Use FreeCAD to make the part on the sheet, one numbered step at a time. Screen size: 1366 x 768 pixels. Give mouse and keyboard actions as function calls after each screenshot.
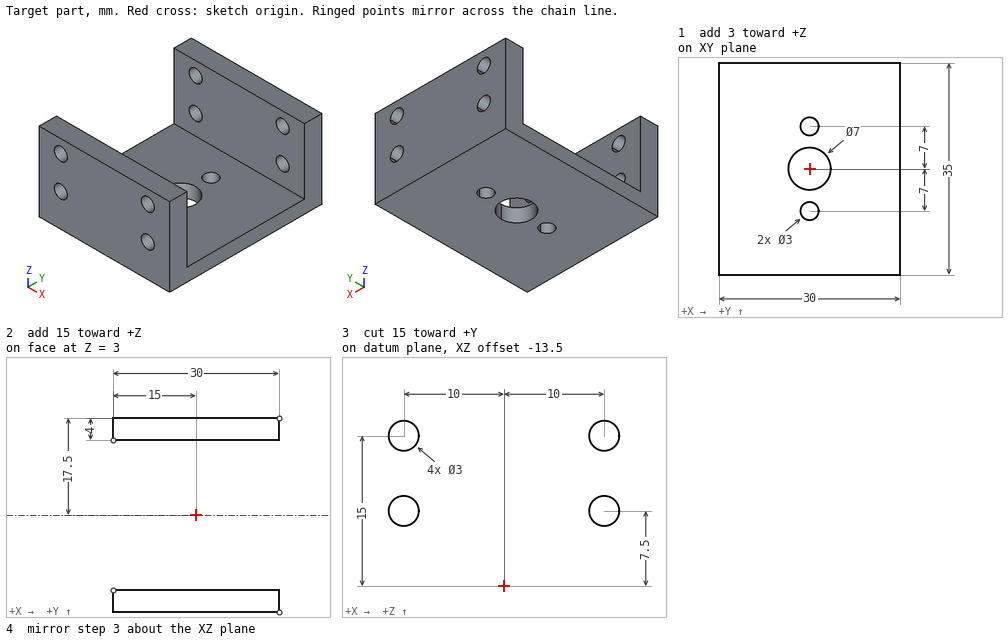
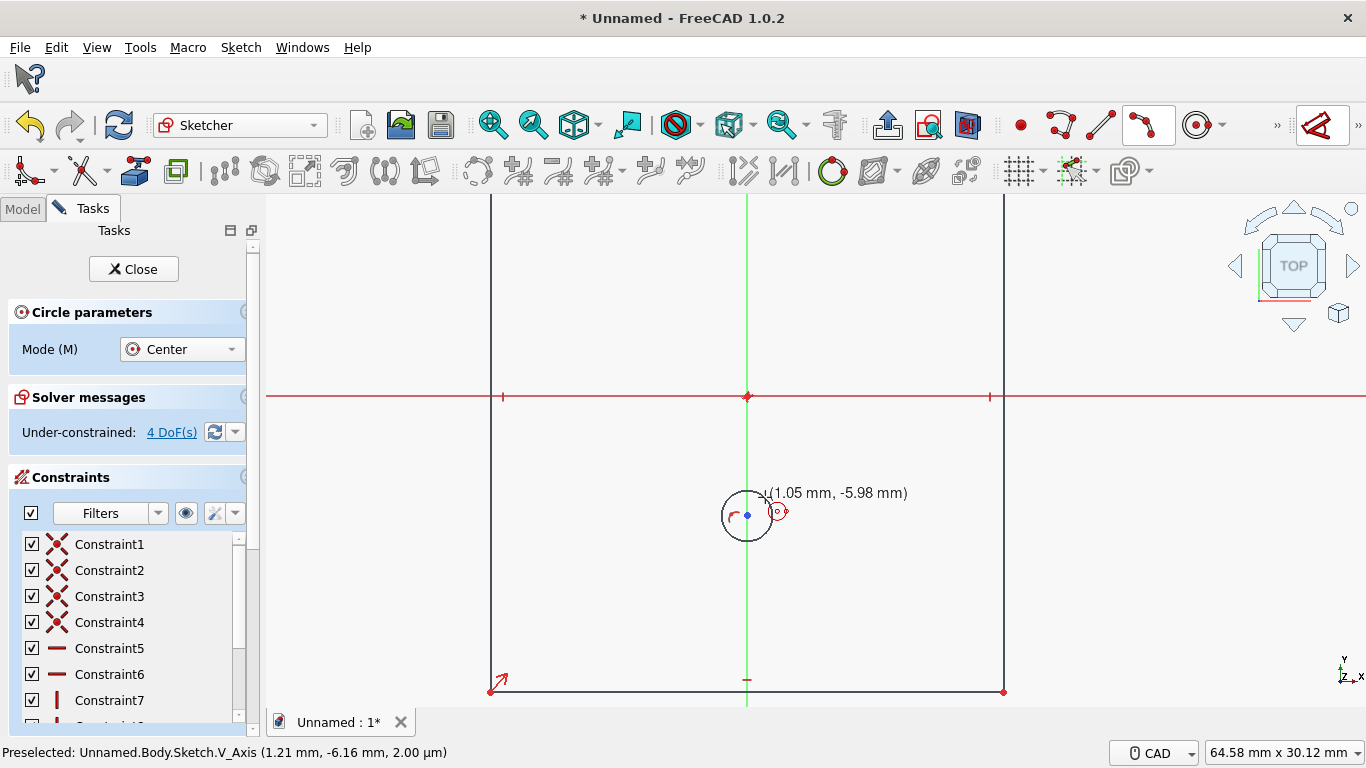
click(747, 396)
click(789, 354)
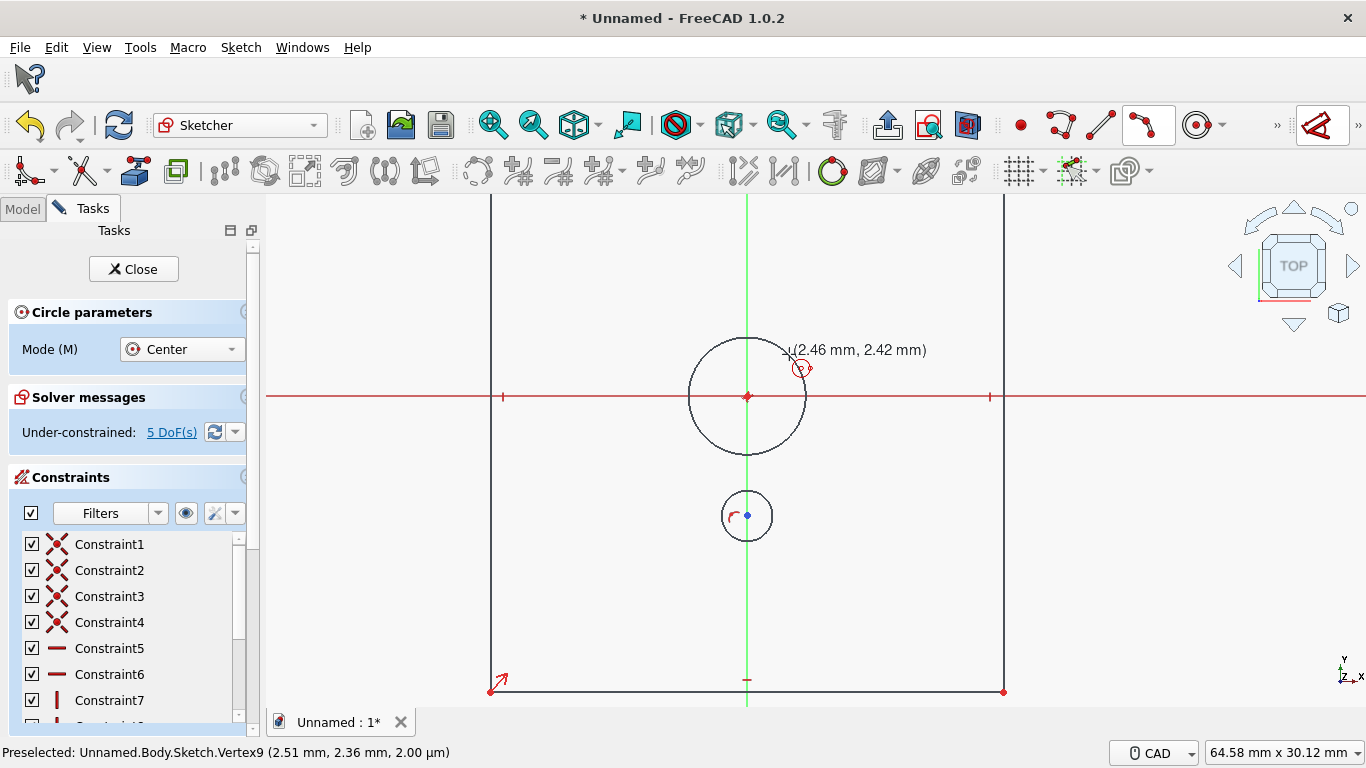
click(747, 277)
click(765, 259)
key(Escape)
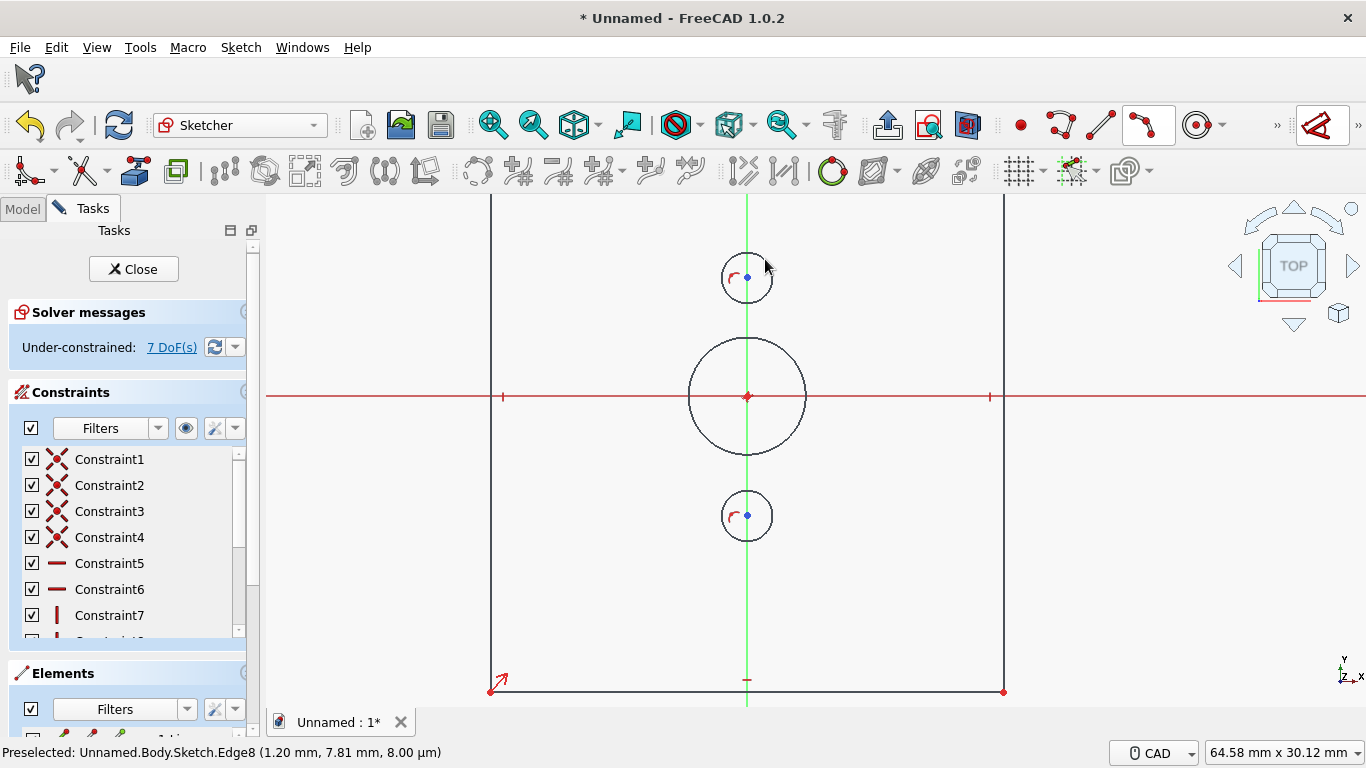
click(765, 498)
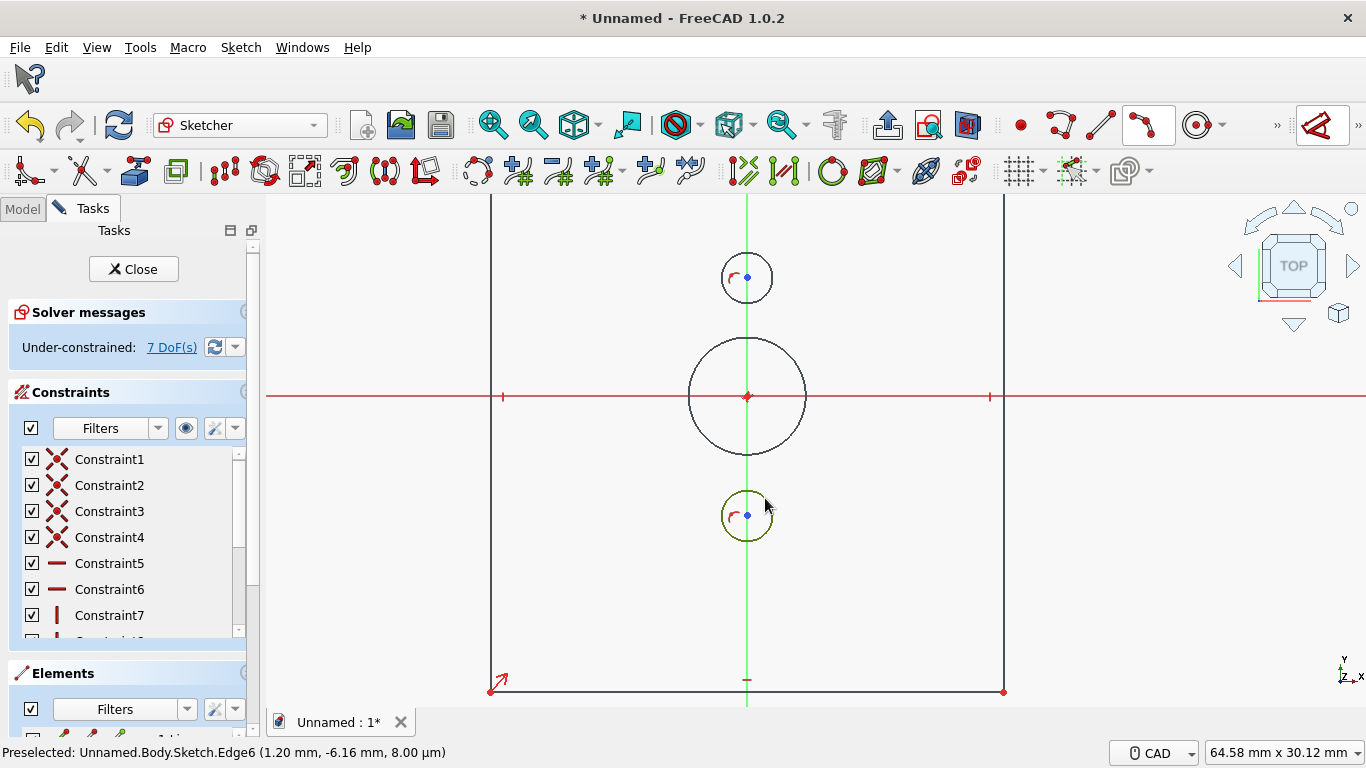
click(765, 260)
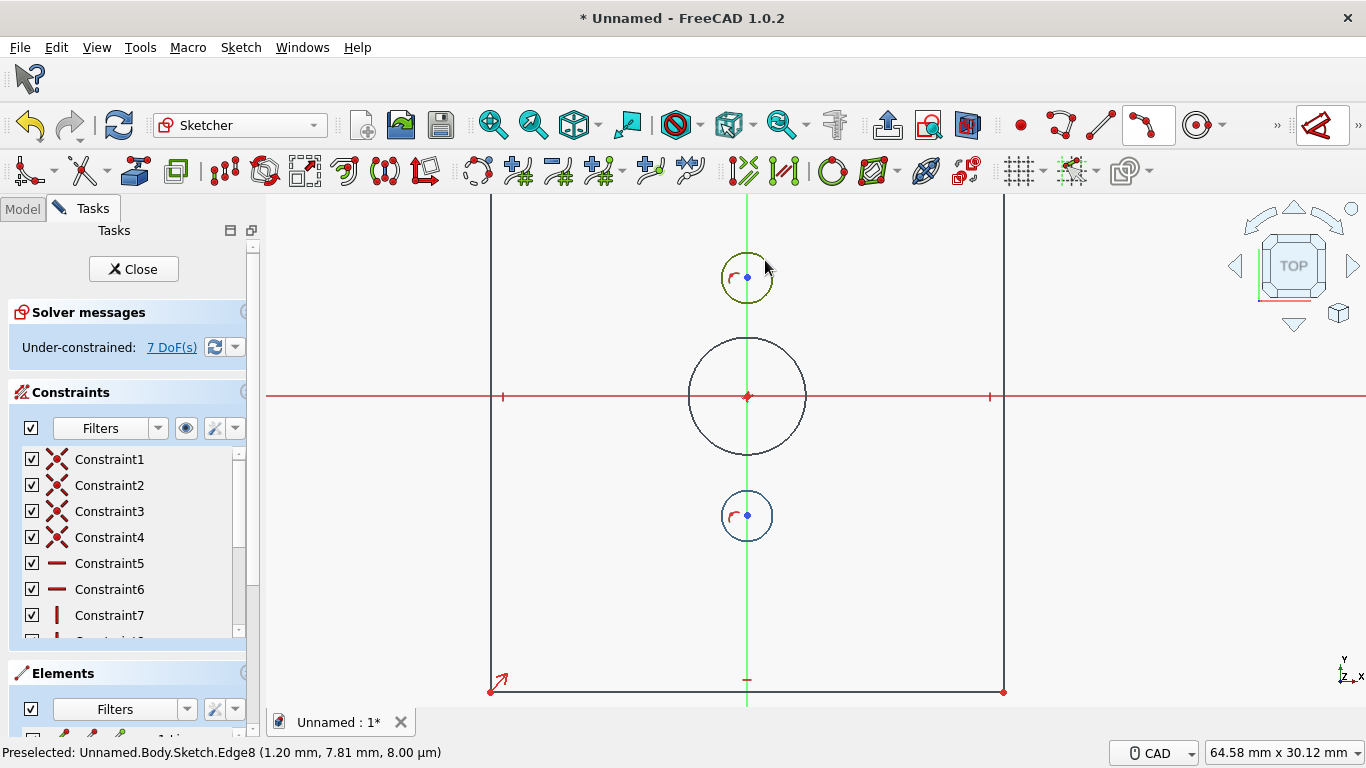
key(e)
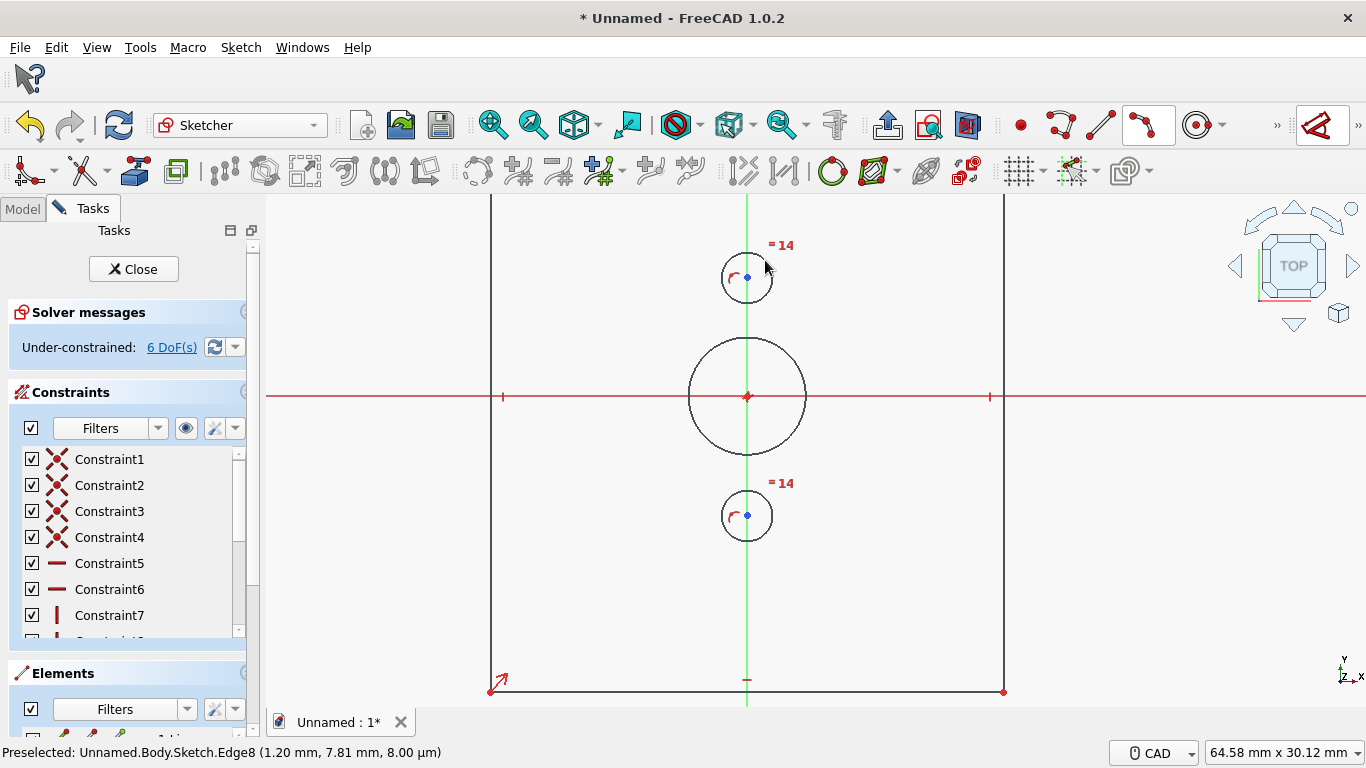
click(1316, 126)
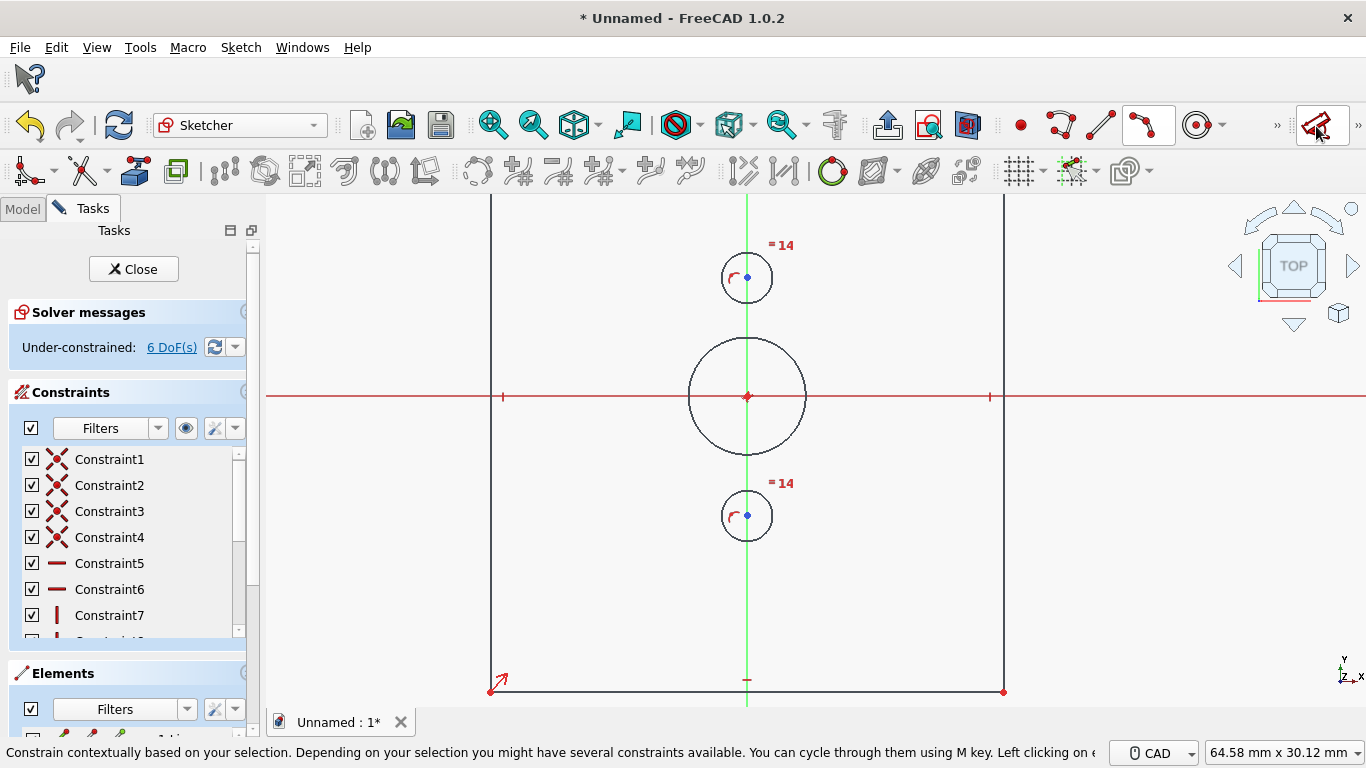
click(765, 498)
click(788, 475)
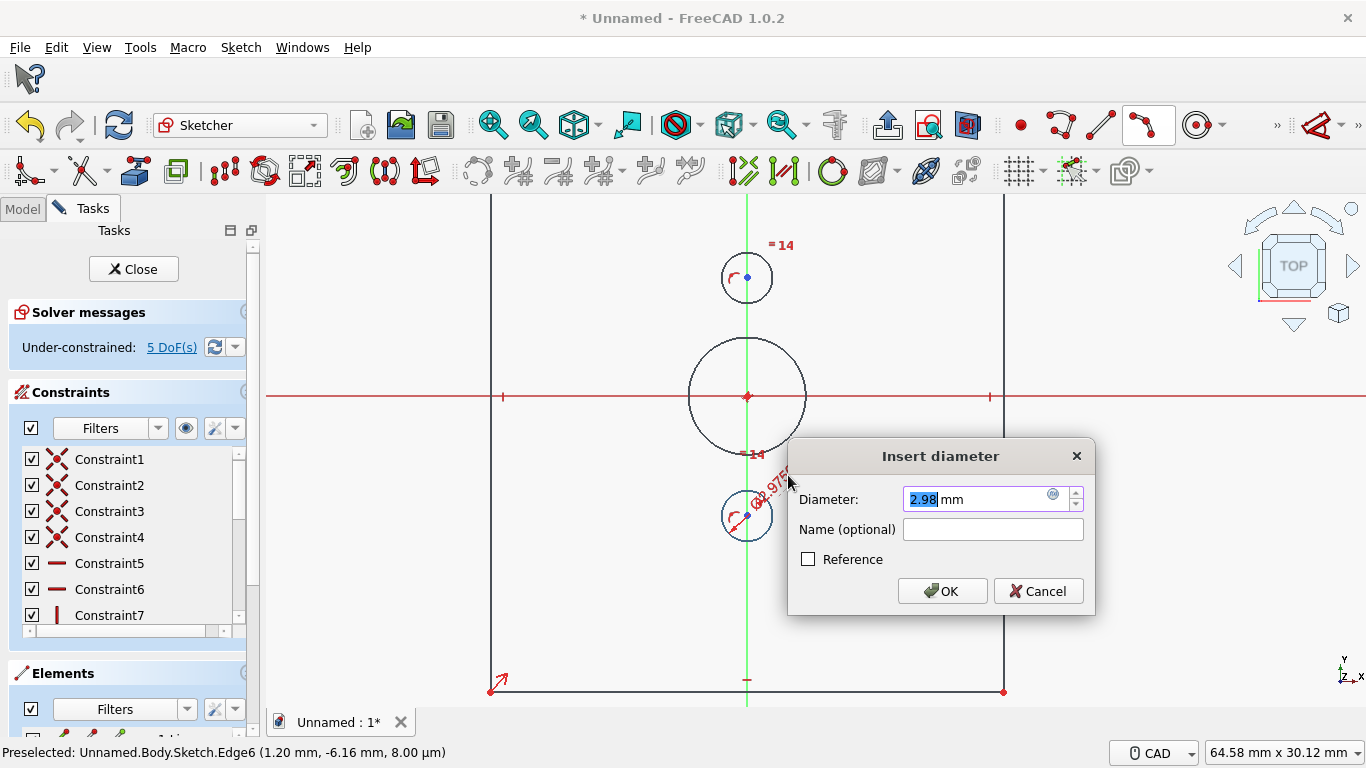
text(3)
key(Return)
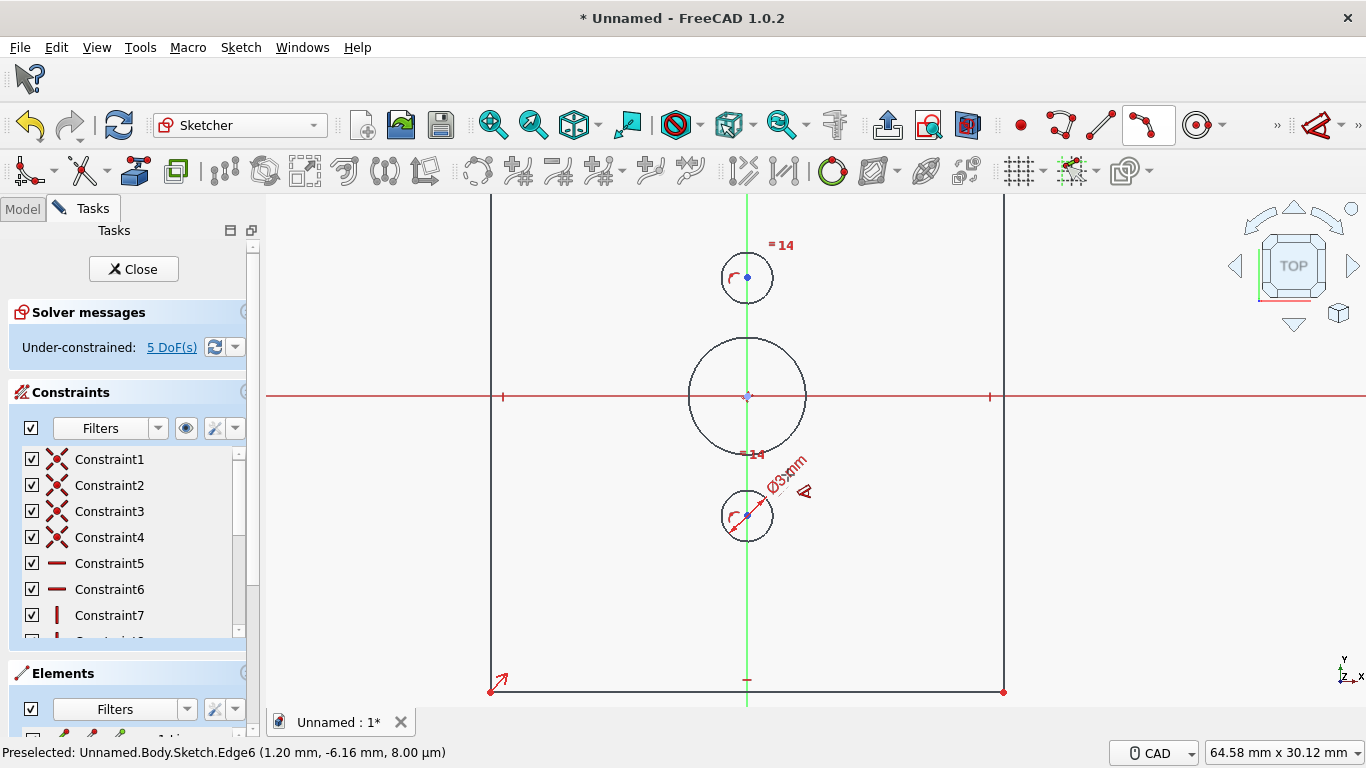
click(789, 355)
click(812, 333)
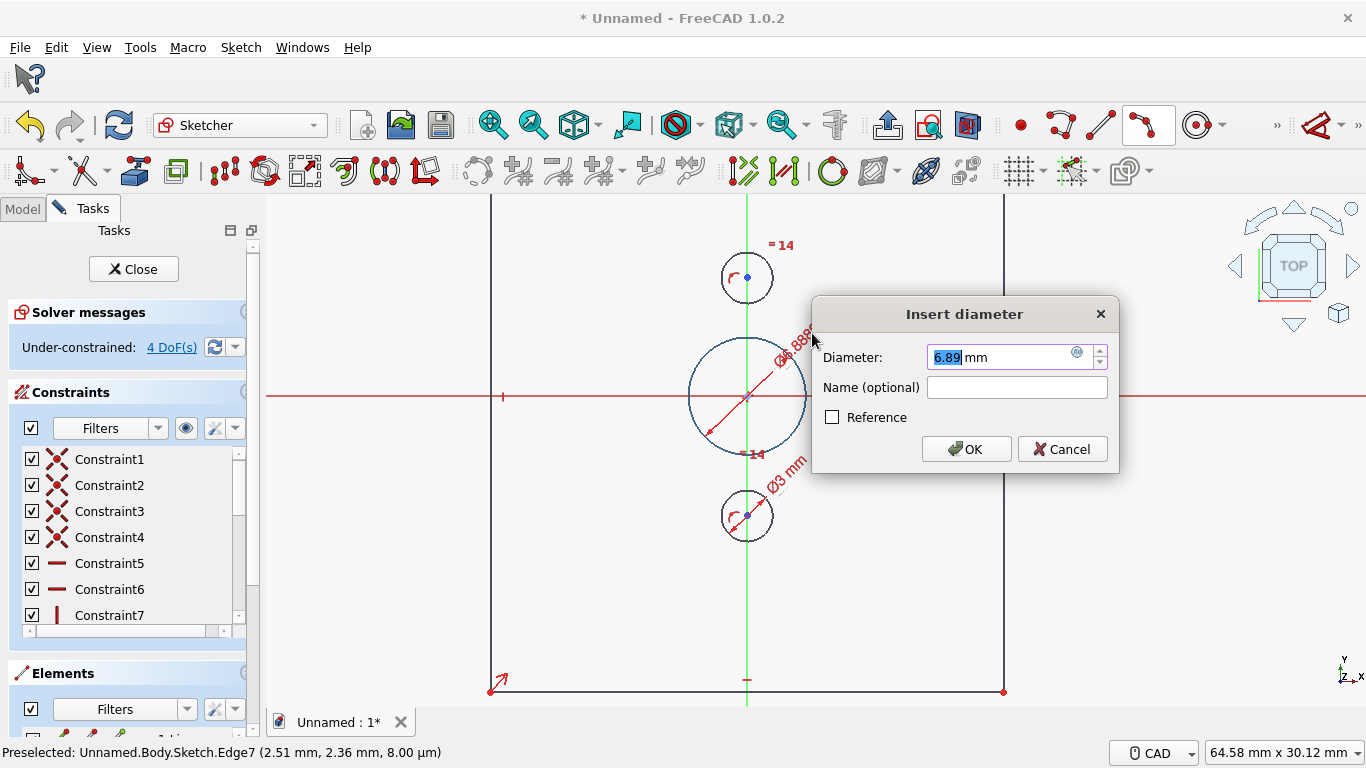
text(7)
key(Return)